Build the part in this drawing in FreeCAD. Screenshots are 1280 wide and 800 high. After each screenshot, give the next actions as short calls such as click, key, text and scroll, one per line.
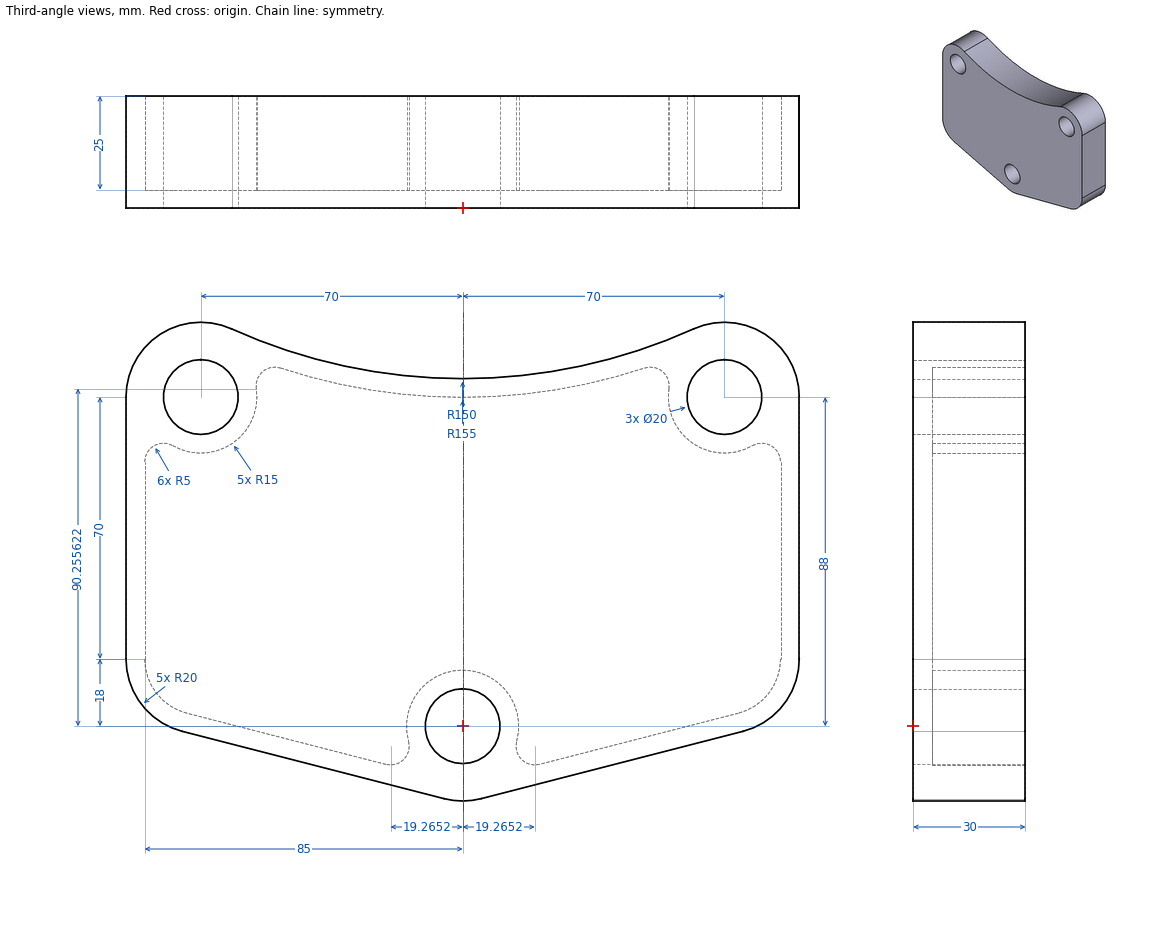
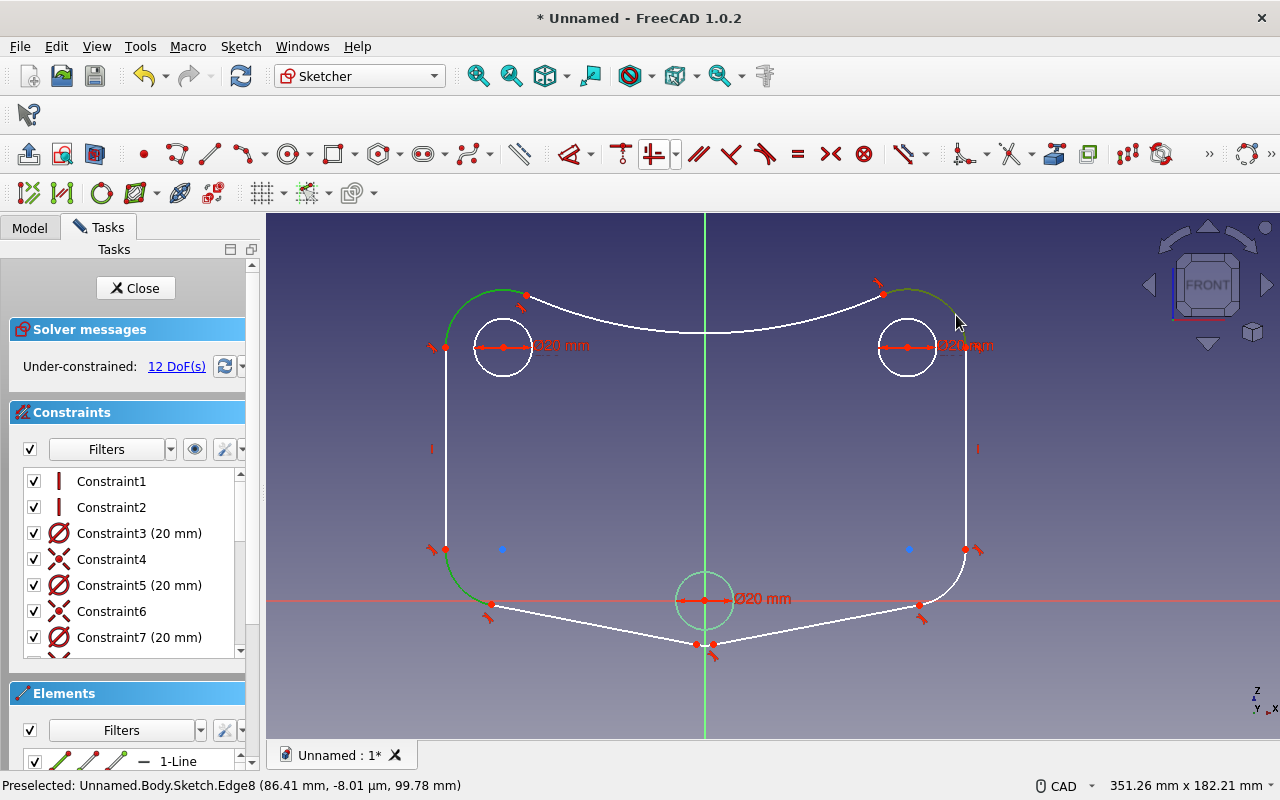
click(961, 572)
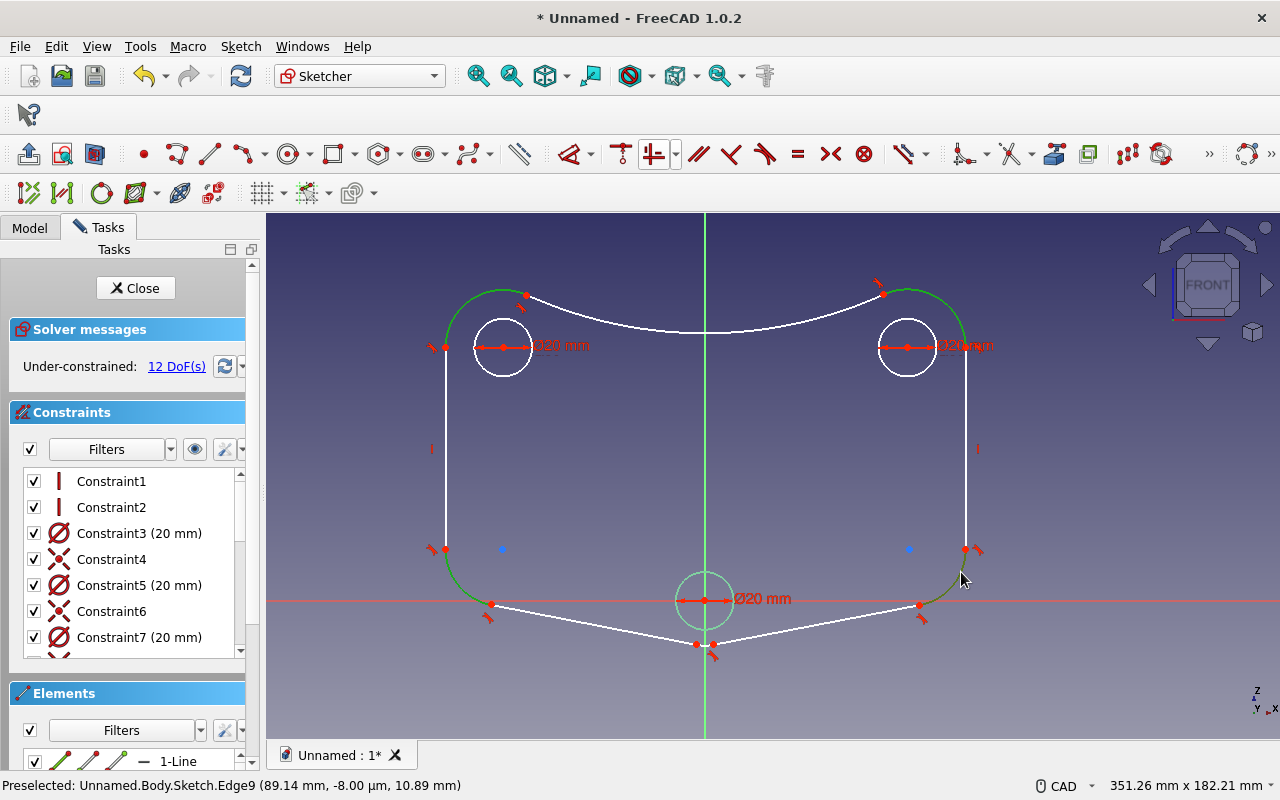
scroll(705, 646, up, 3)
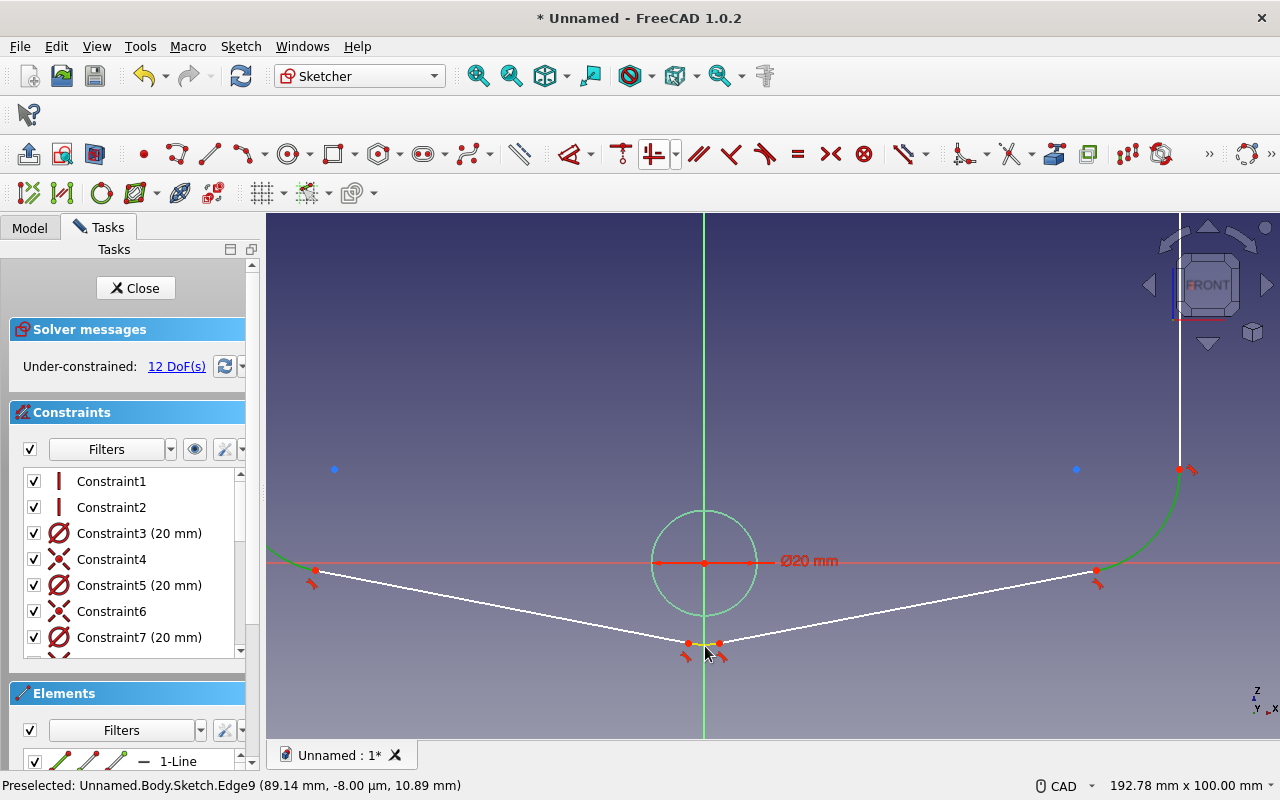
click(704, 645)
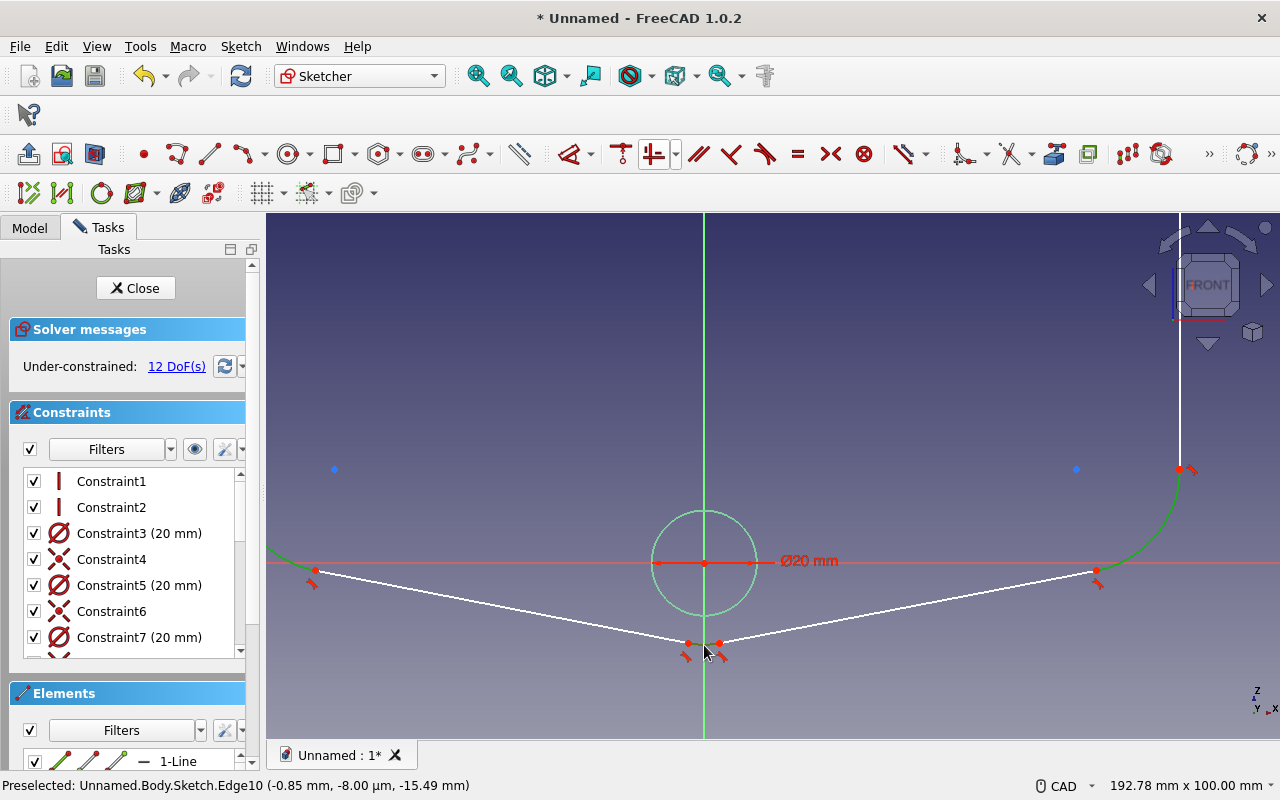
click(798, 154)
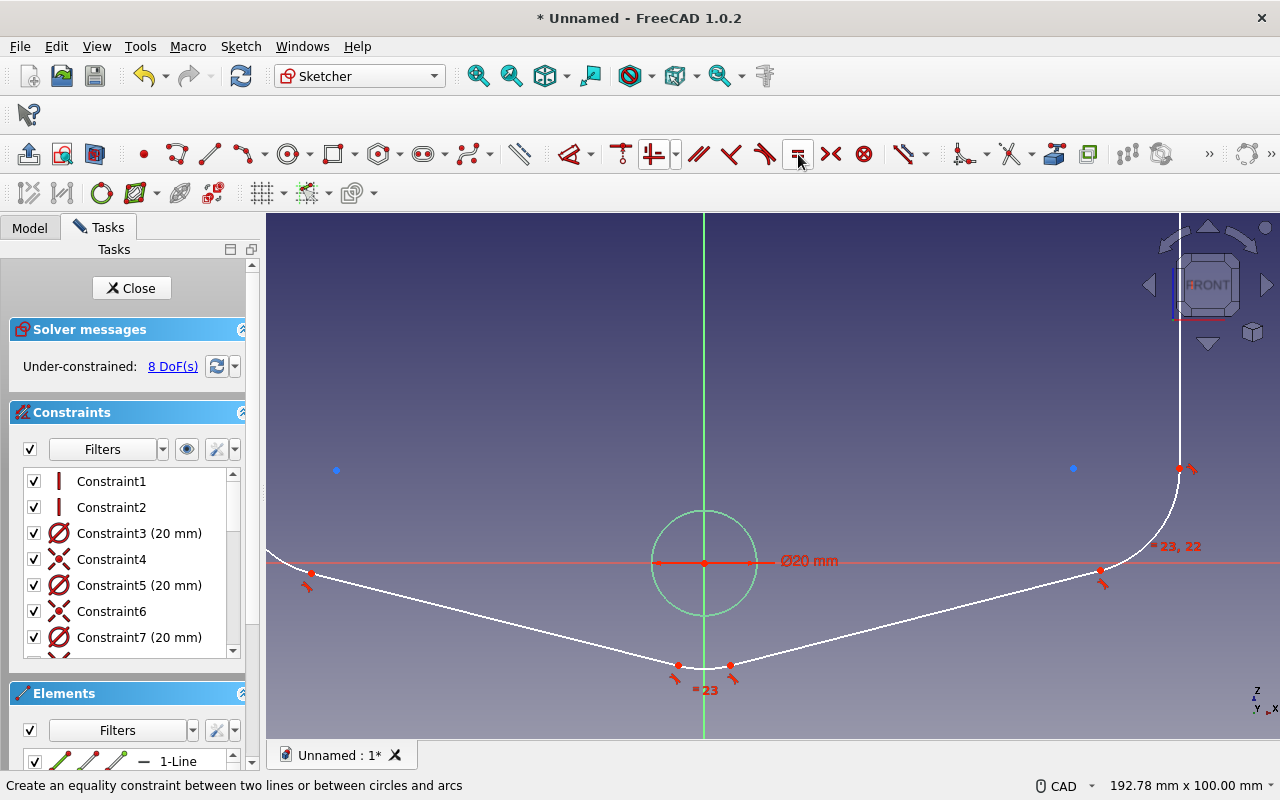
scroll(705, 646, down, 3)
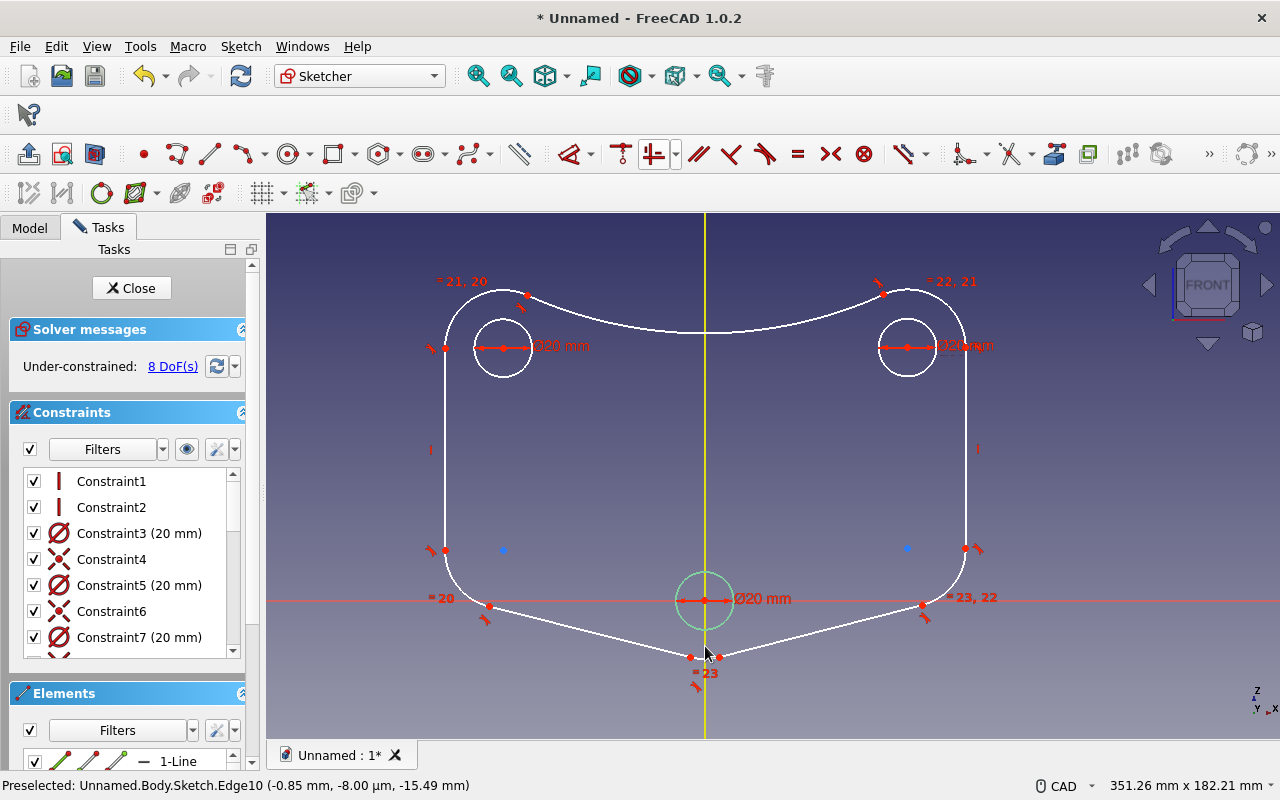
scroll(704, 636, down, 4)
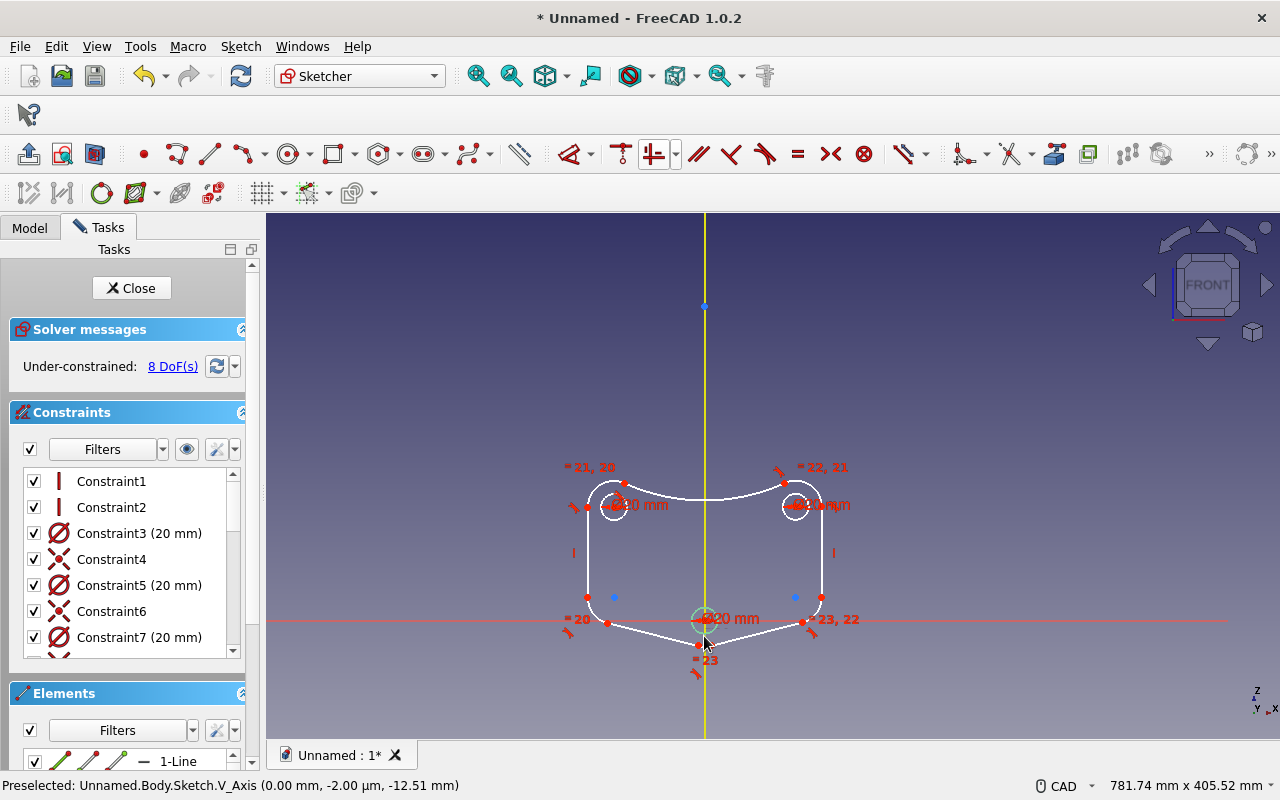
click(705, 306)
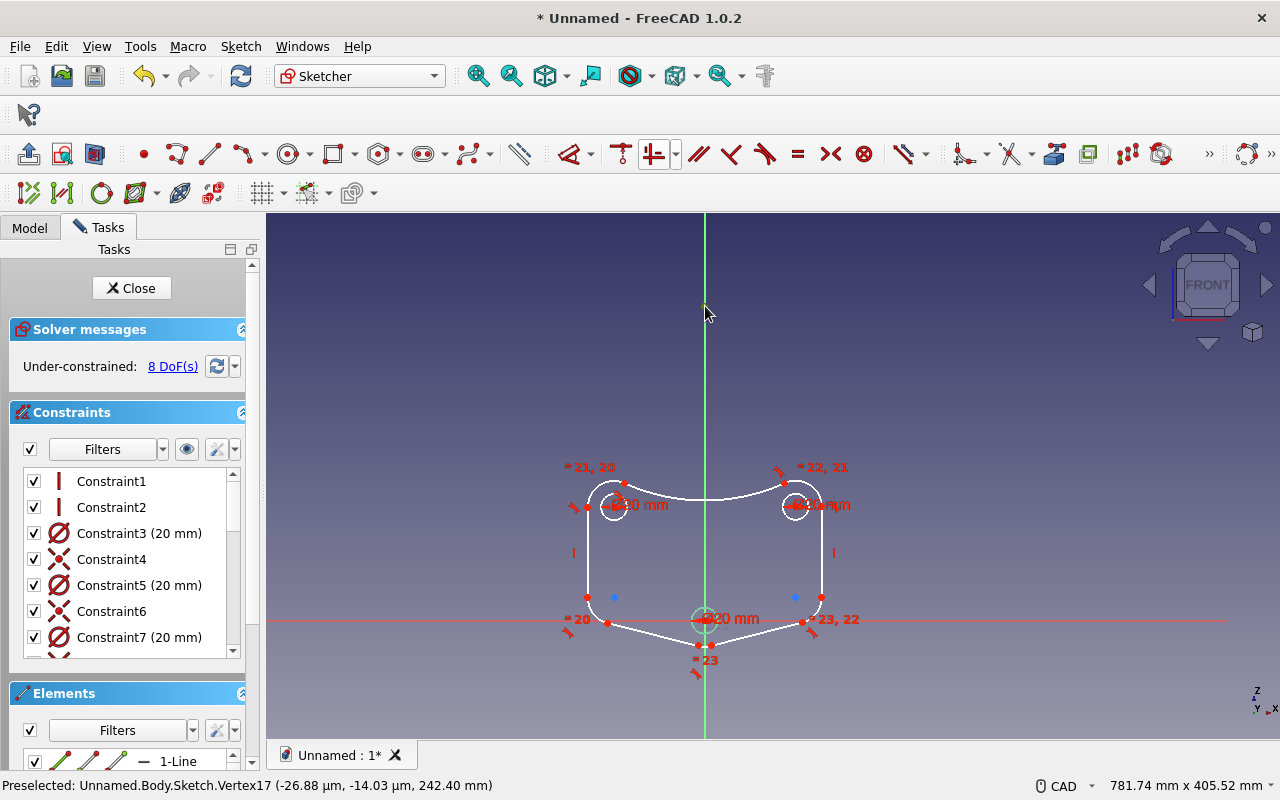
click(705, 577)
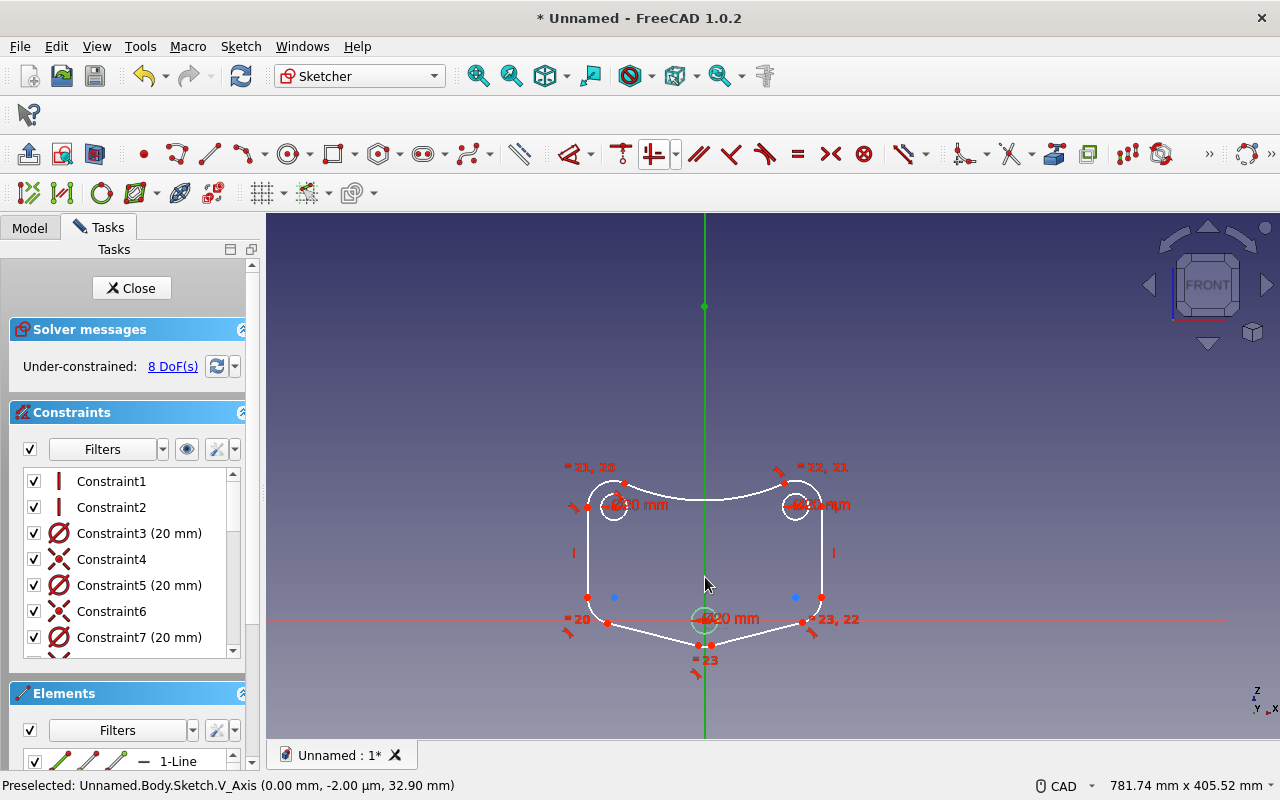
click(621, 154)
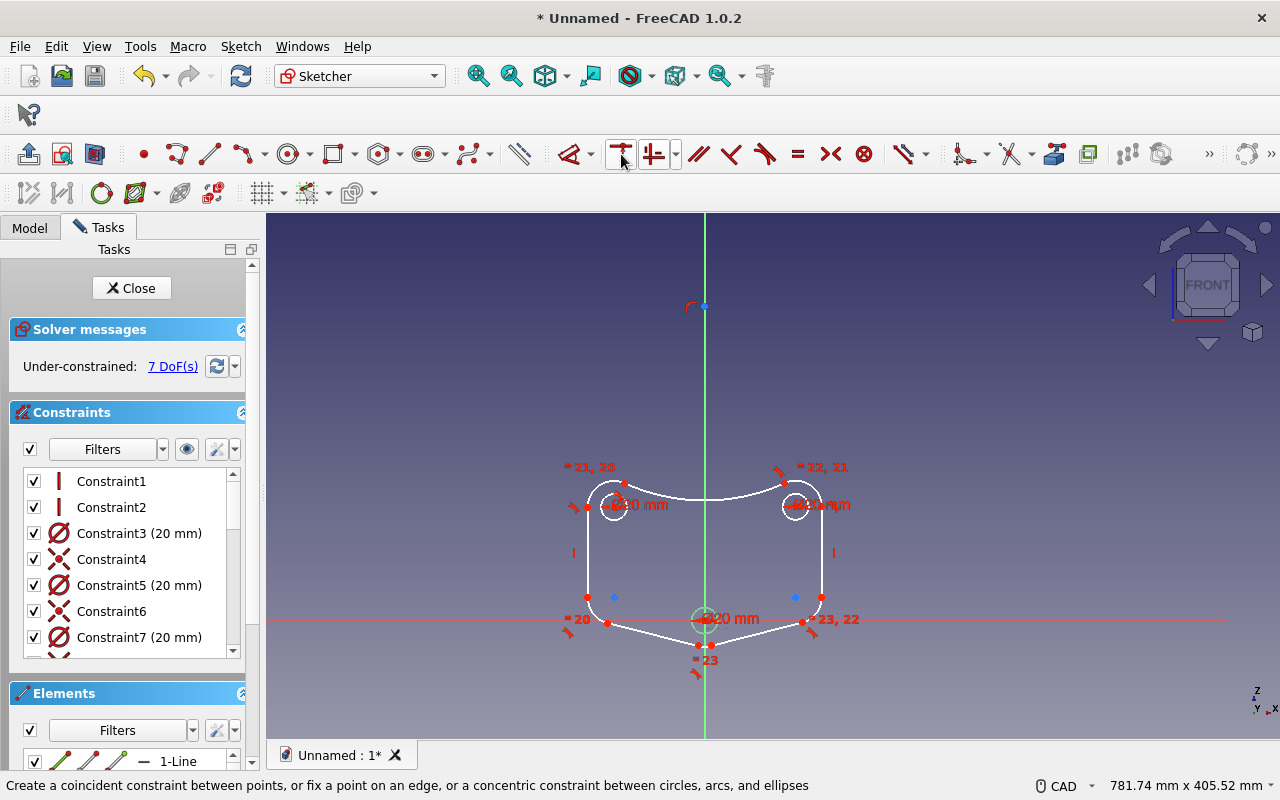
click(614, 598)